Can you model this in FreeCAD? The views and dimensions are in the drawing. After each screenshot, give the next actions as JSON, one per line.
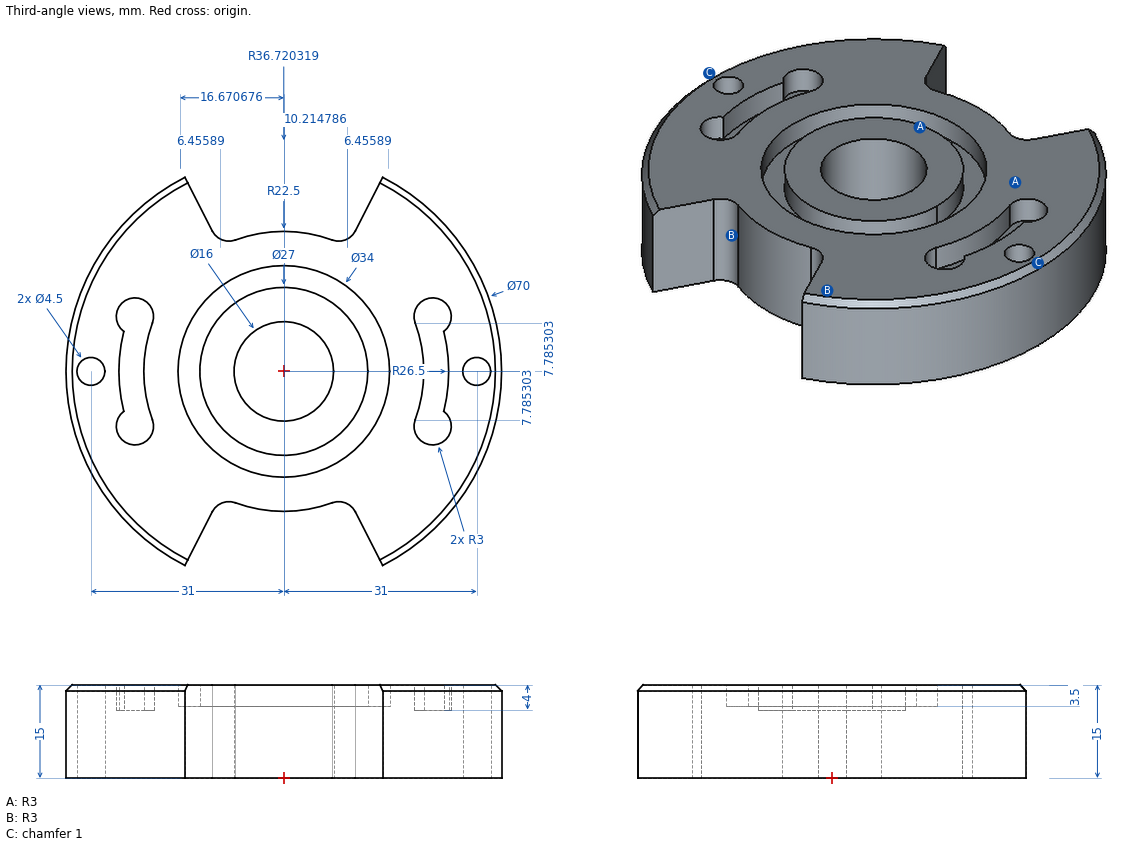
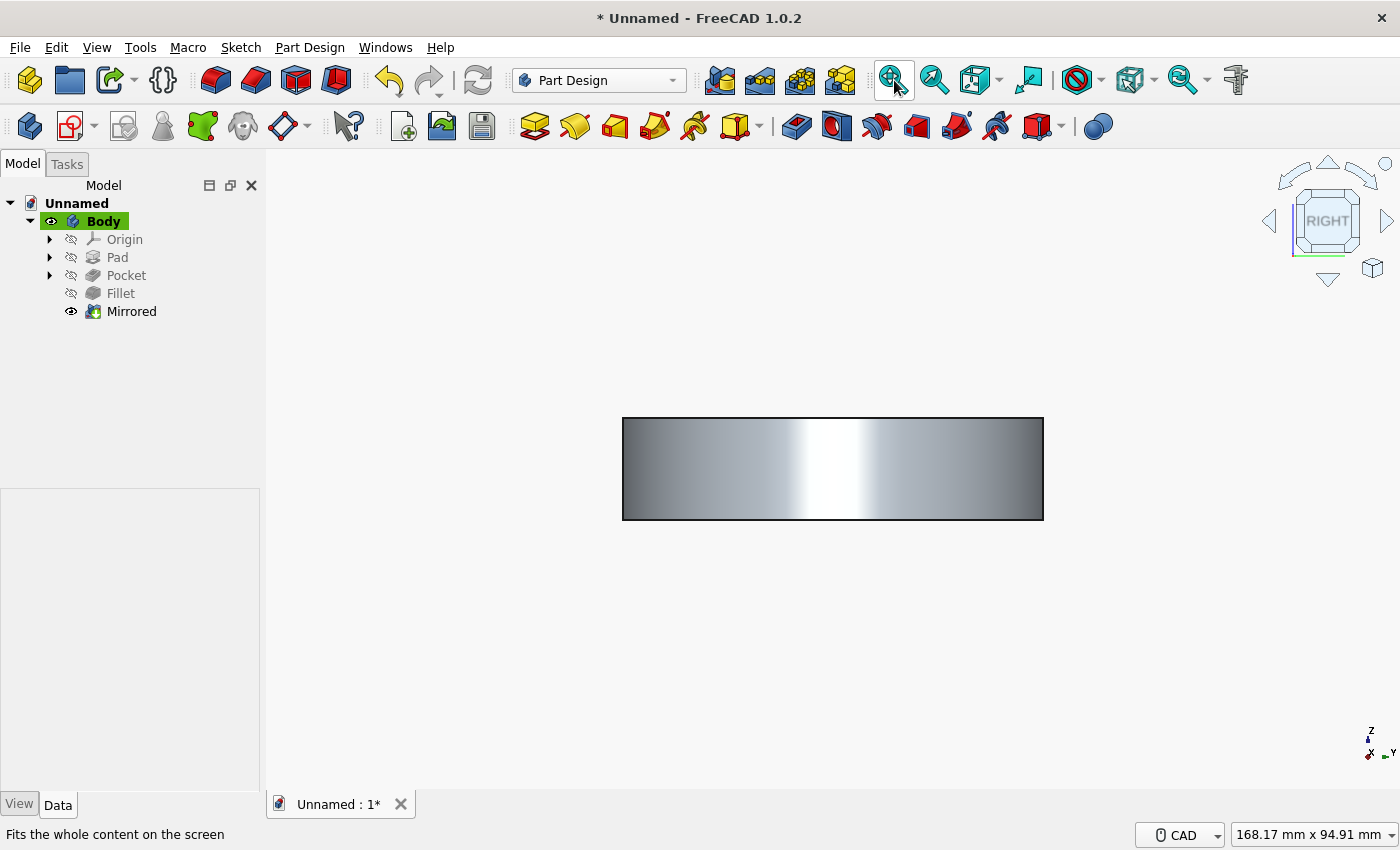
{"action": "key", "text": "5"}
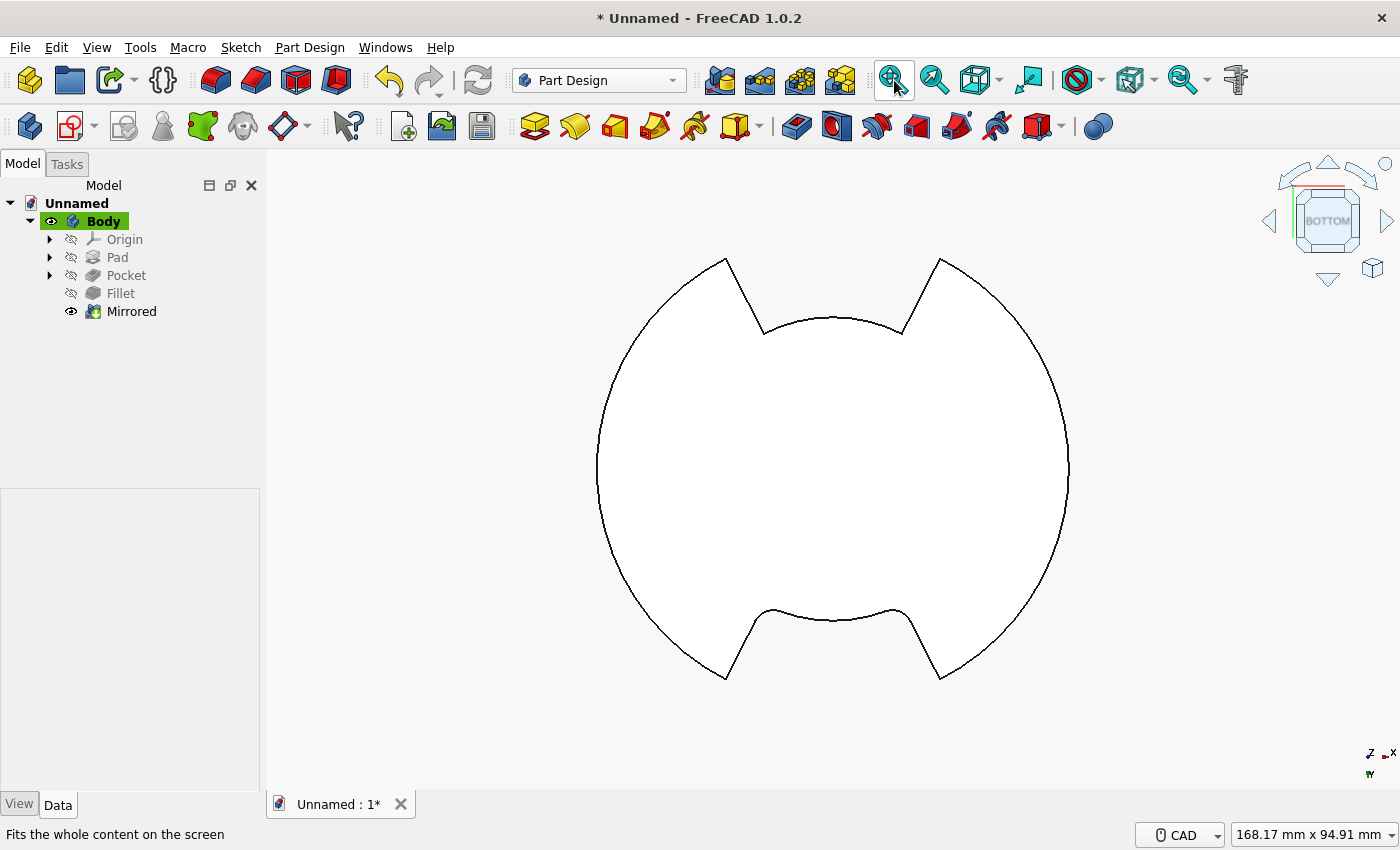
{"action": "key", "text": "4"}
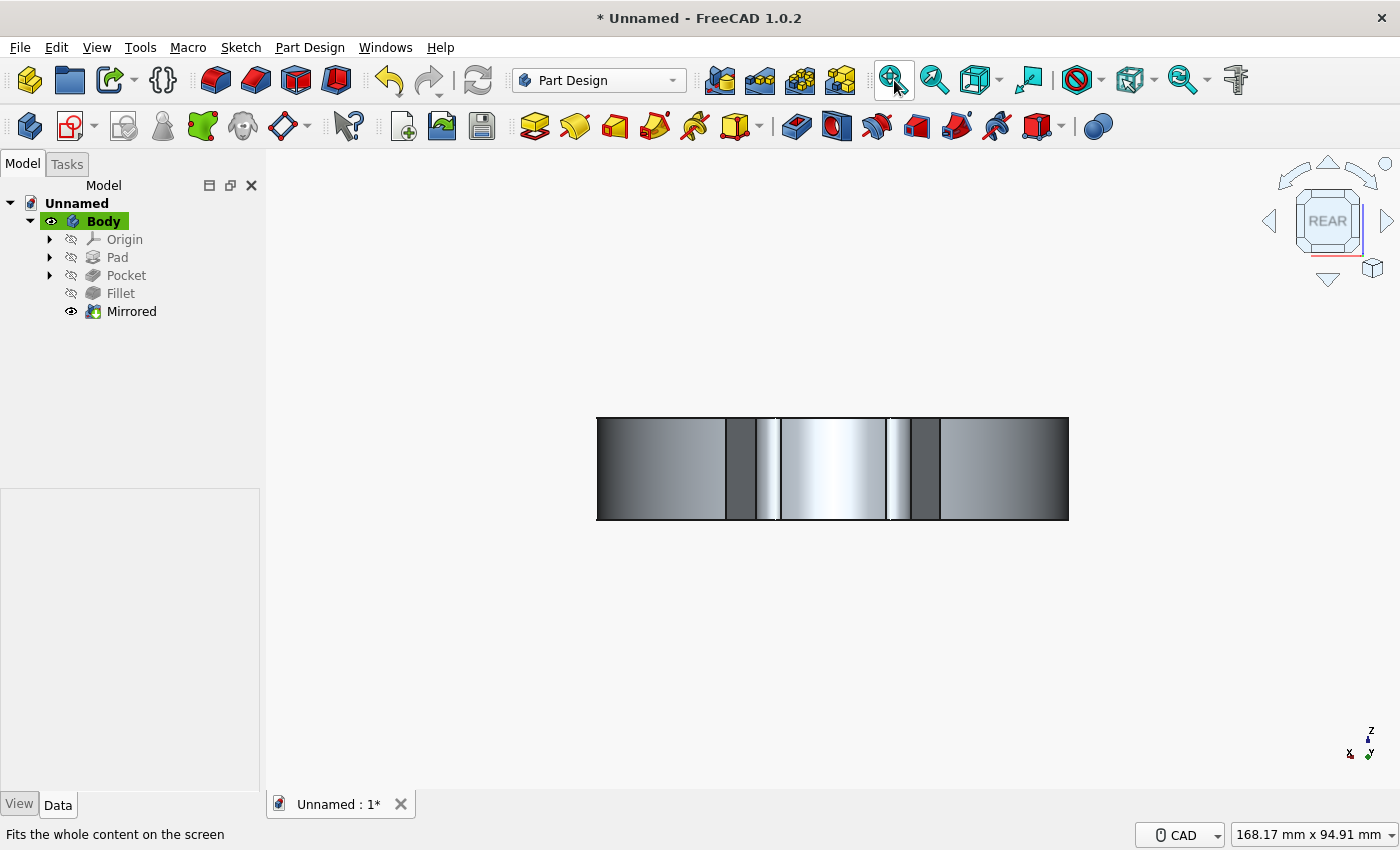
{"action": "left_click", "coordinate": [894, 80]}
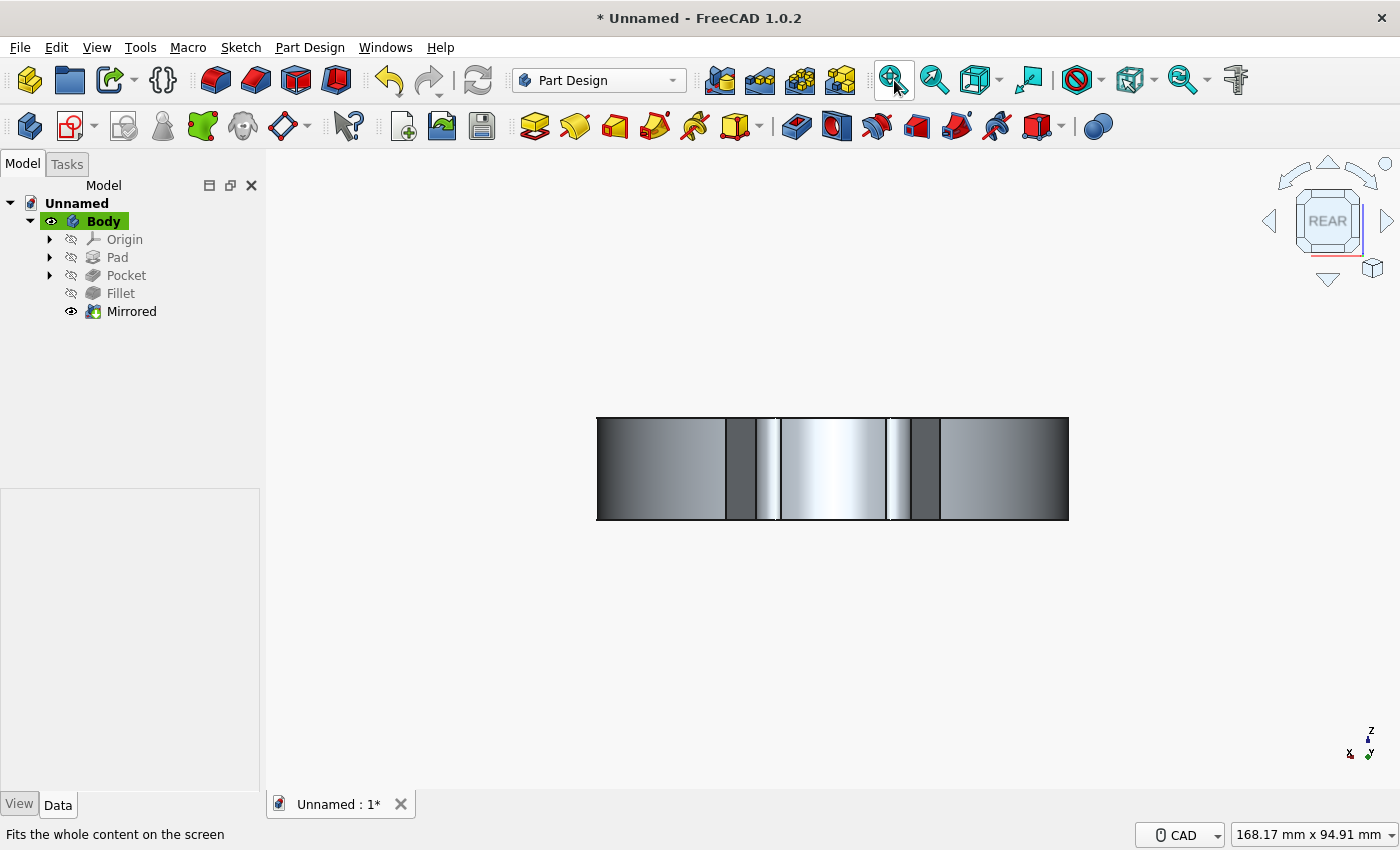
{"action": "key", "text": "6"}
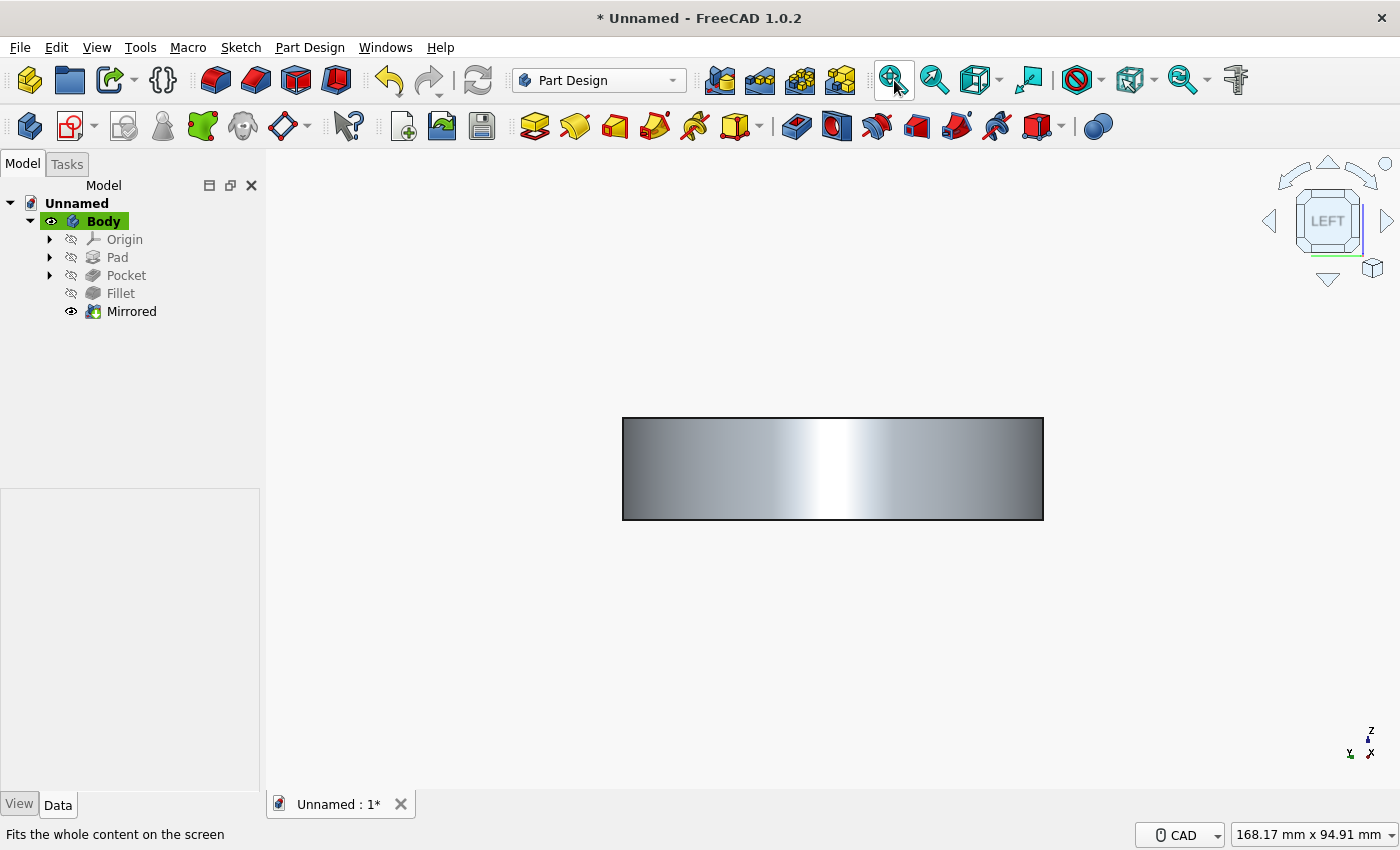
{"action": "key", "text": "v f"}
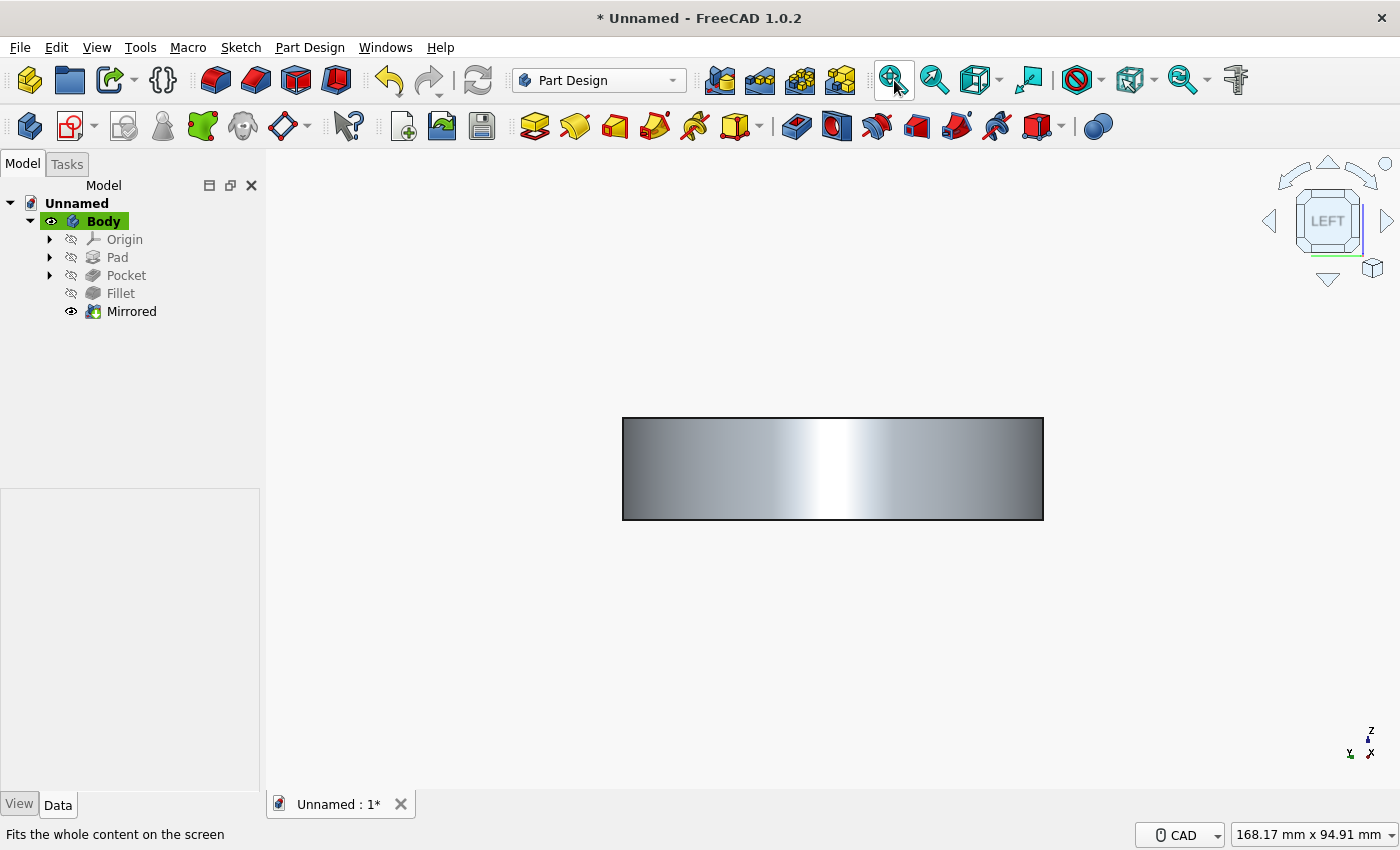
{"action": "key", "text": "v 3"}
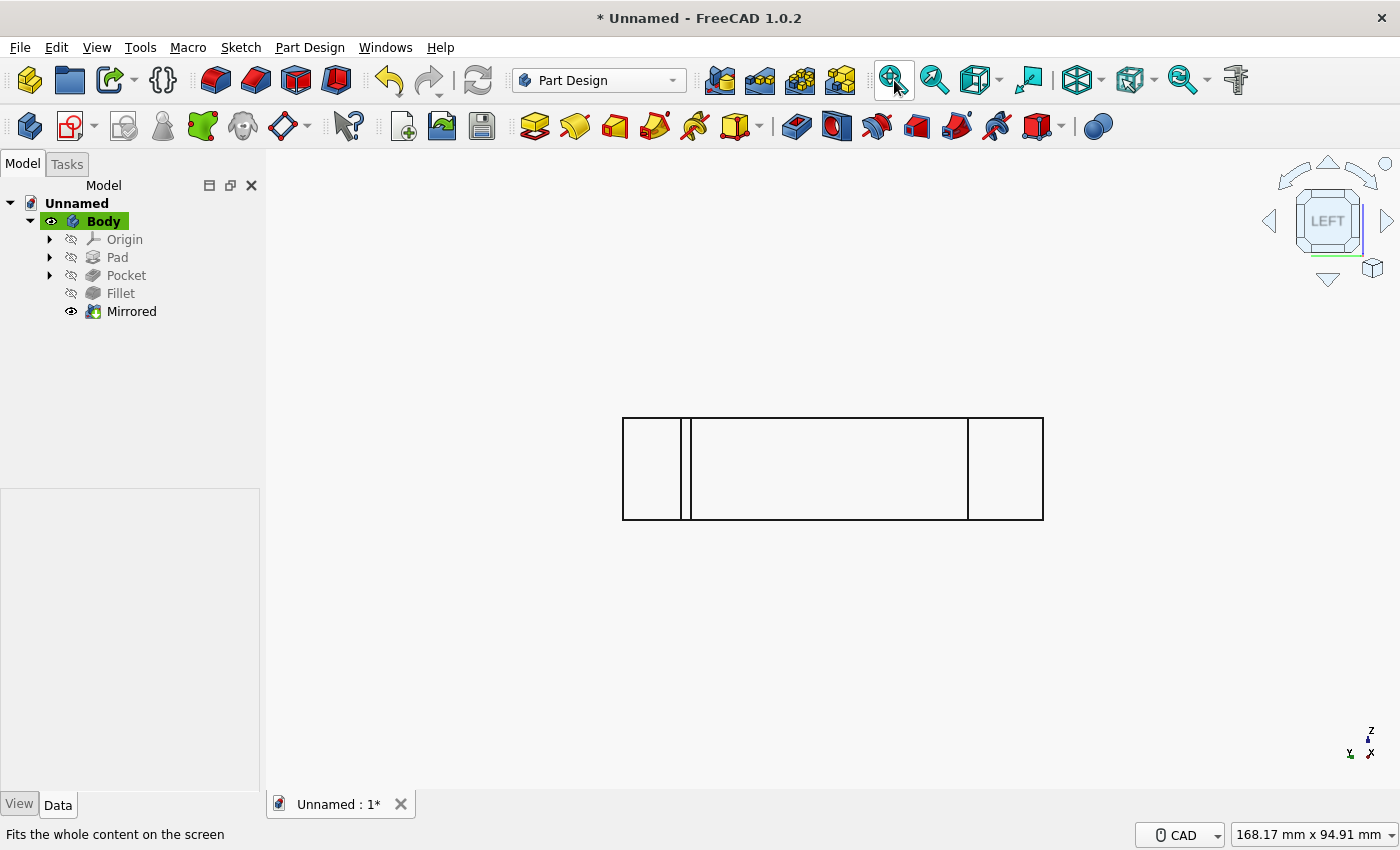
{"action": "key", "text": "0"}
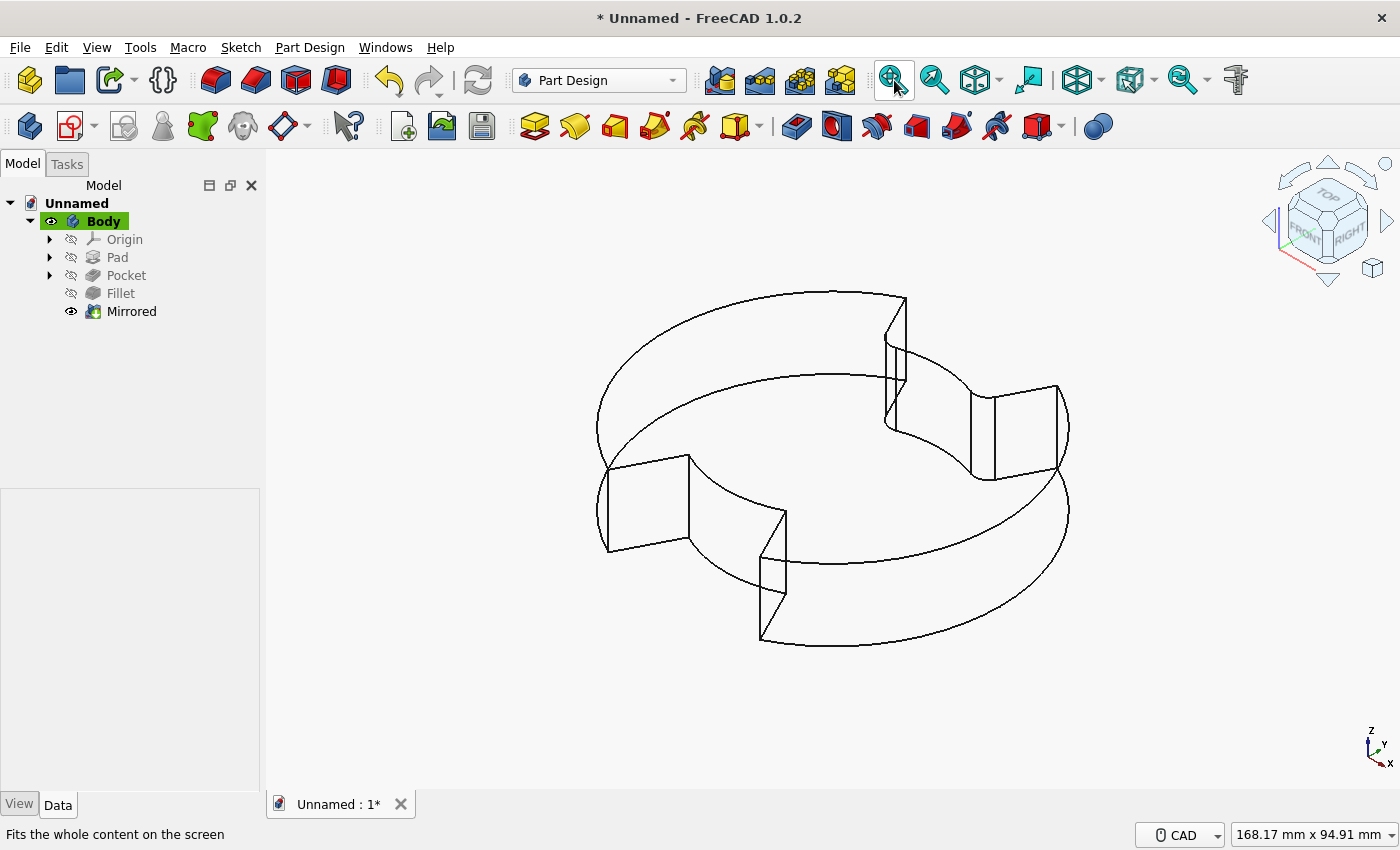
{"action": "left_click", "coordinate": [689, 495]}